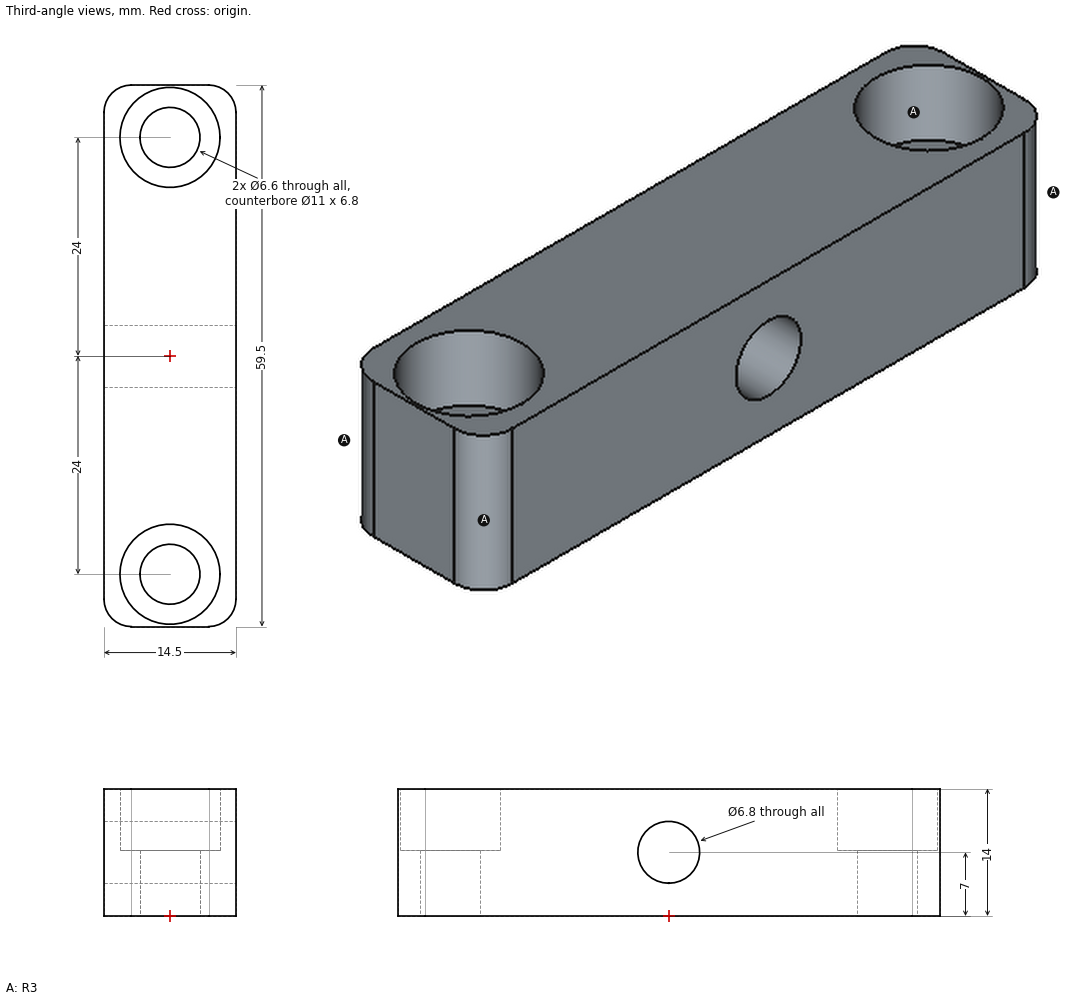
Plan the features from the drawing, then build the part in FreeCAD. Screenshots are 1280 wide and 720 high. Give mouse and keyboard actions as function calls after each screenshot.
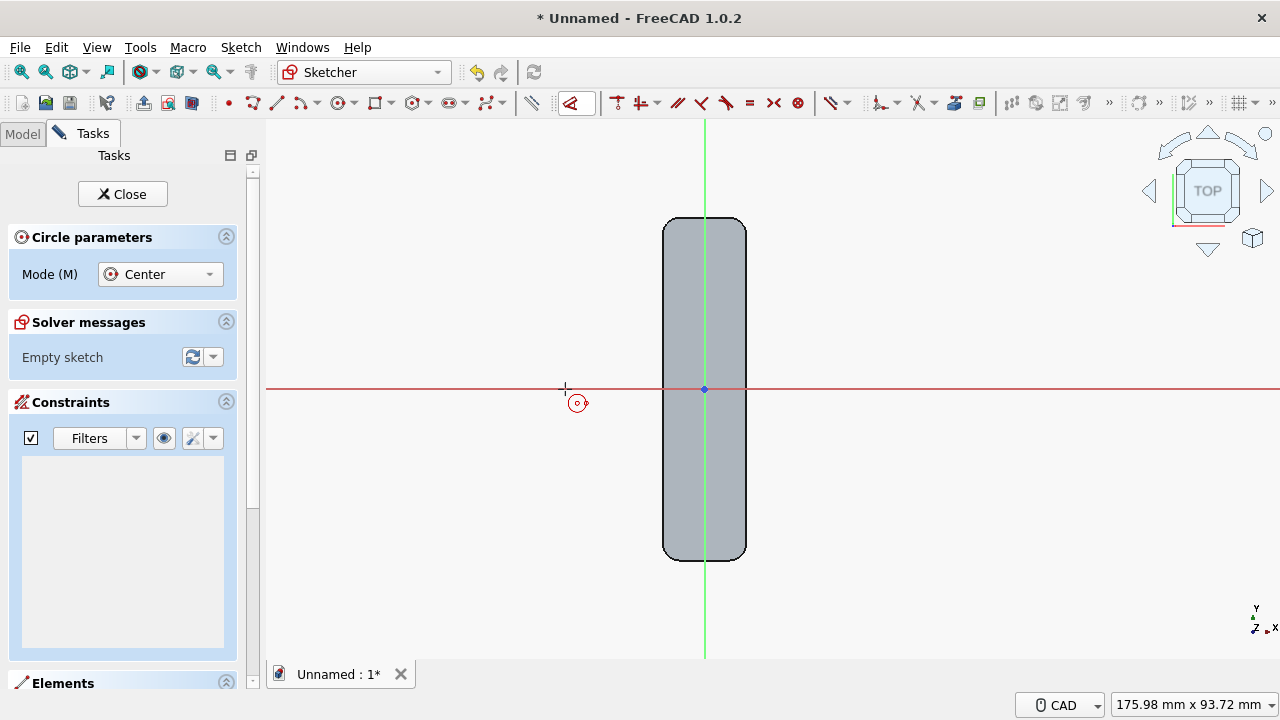
click(705, 251)
move(722, 244)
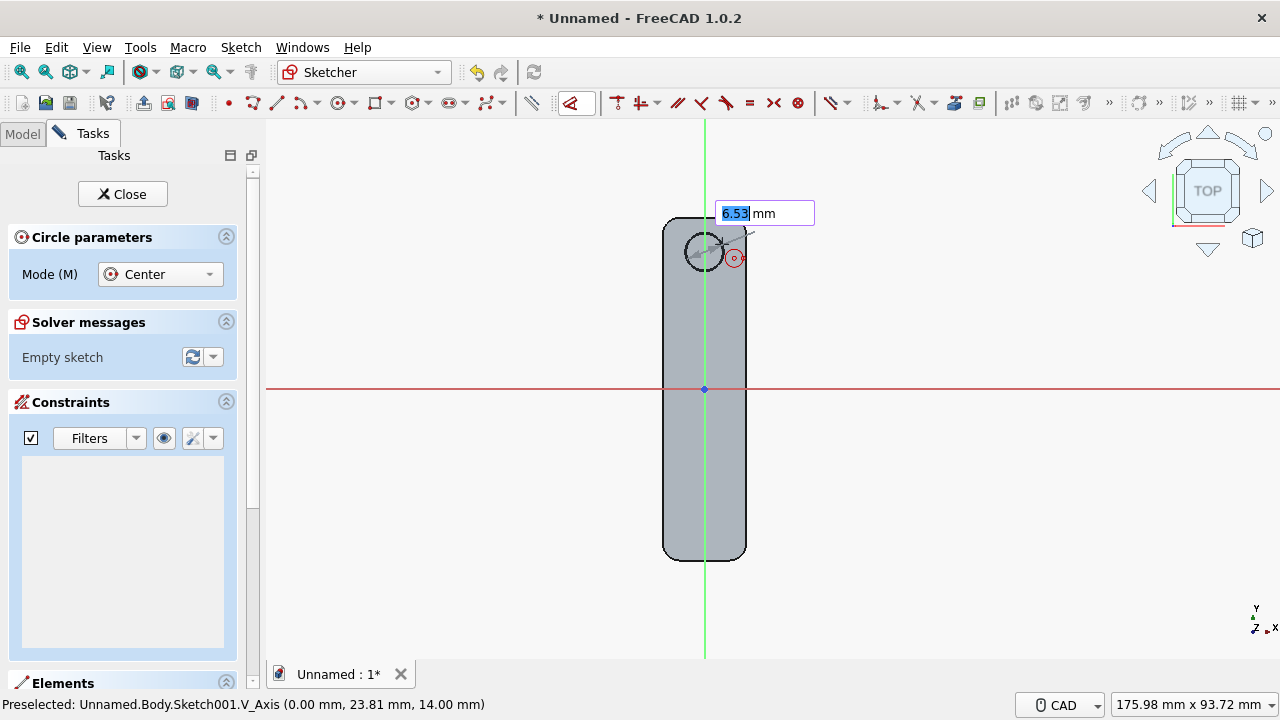
text(6.6)
key(Return)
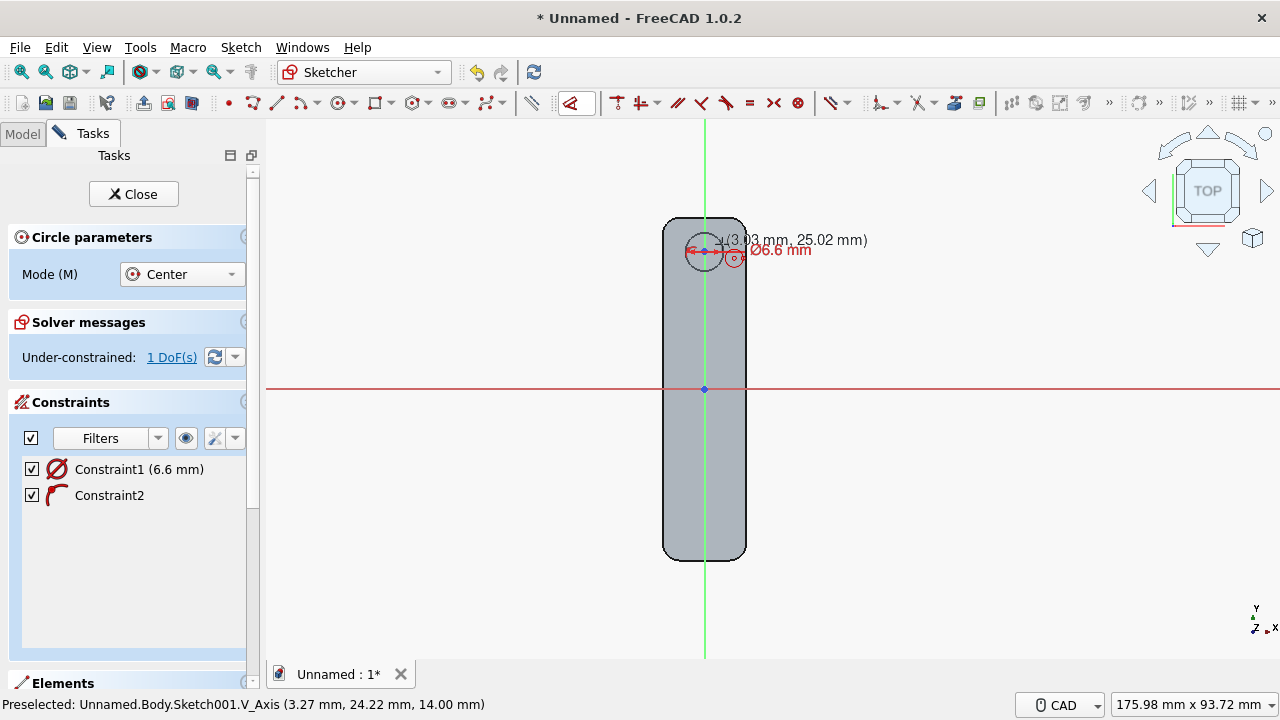
click(705, 527)
move(722, 521)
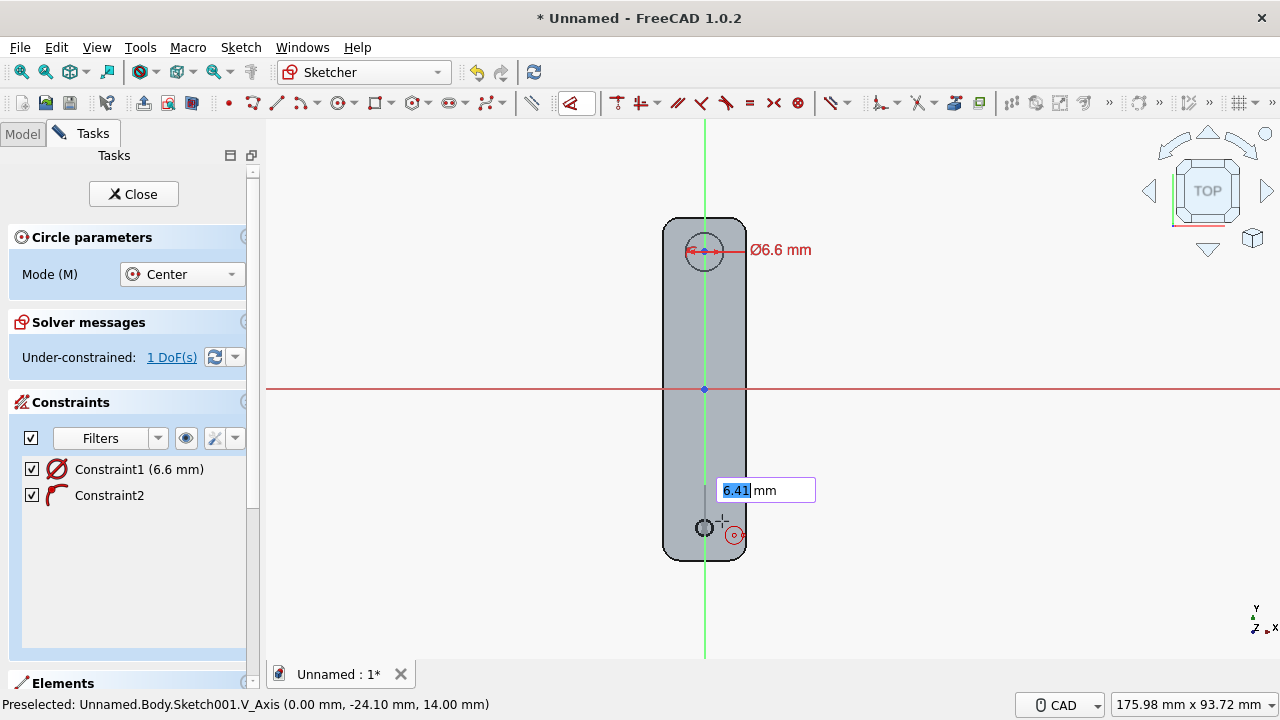
text(6.6)
key(Return)
key(Escape)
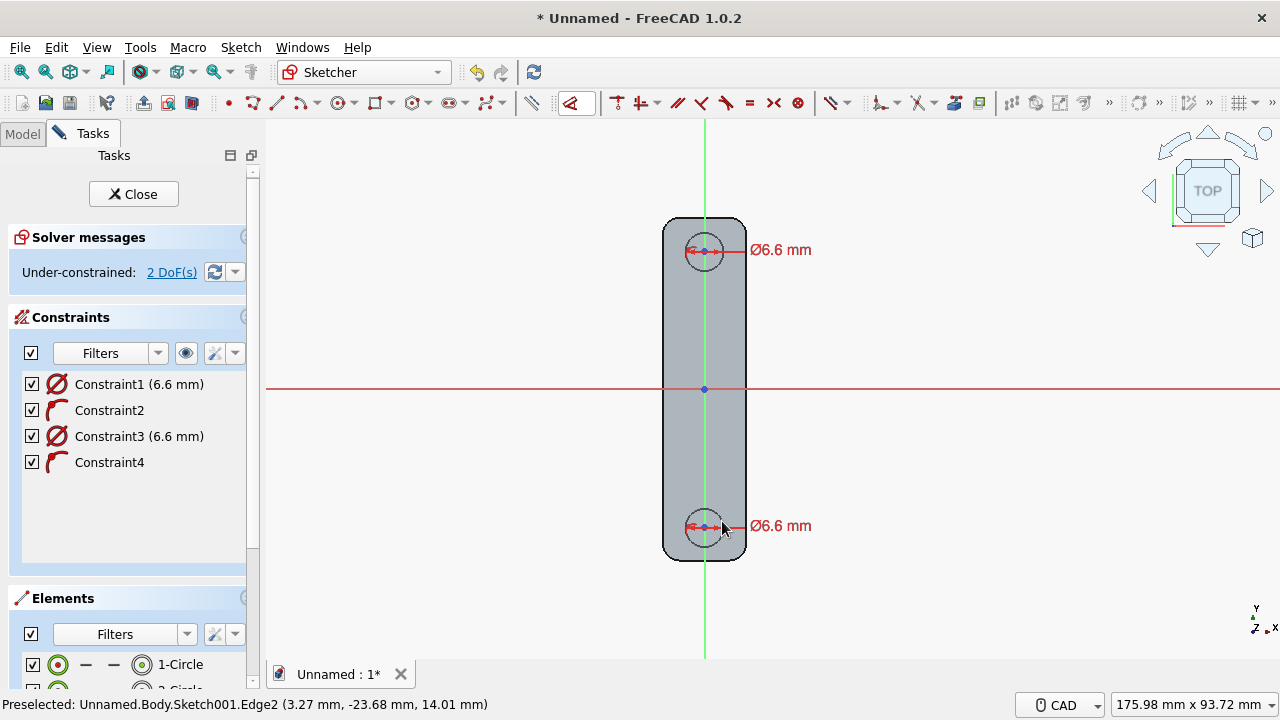
click(705, 252)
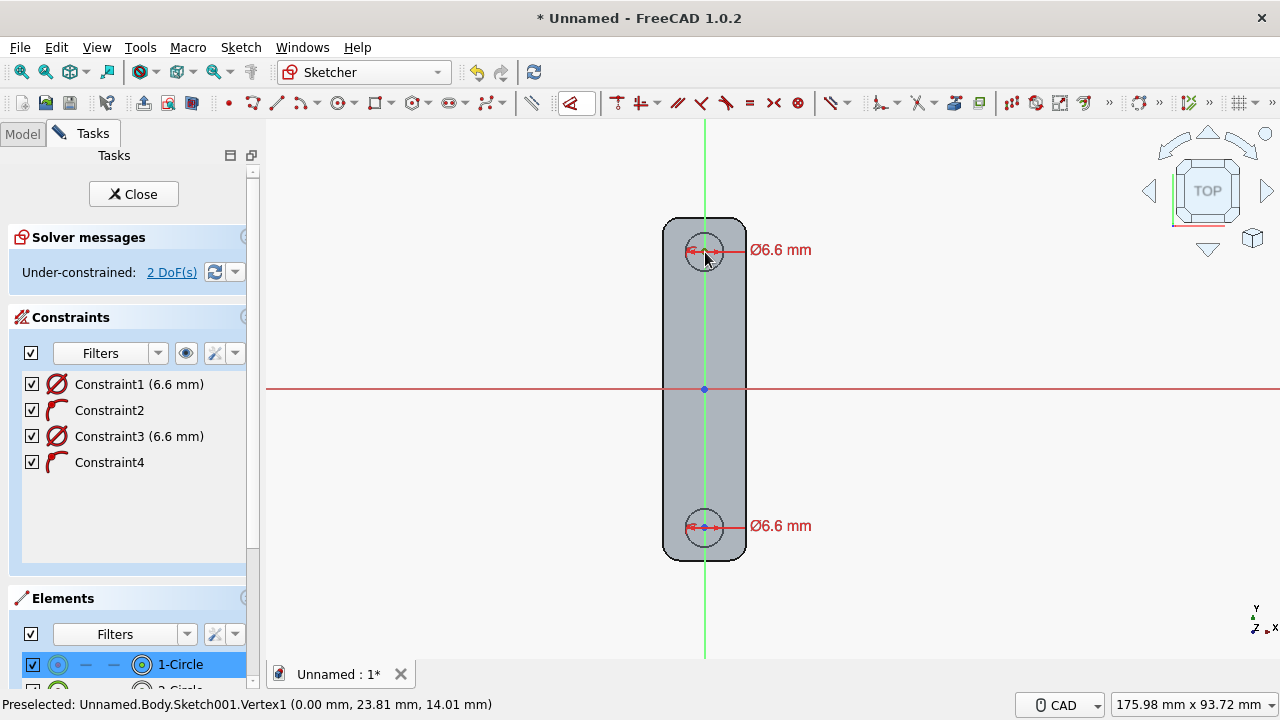
key(i)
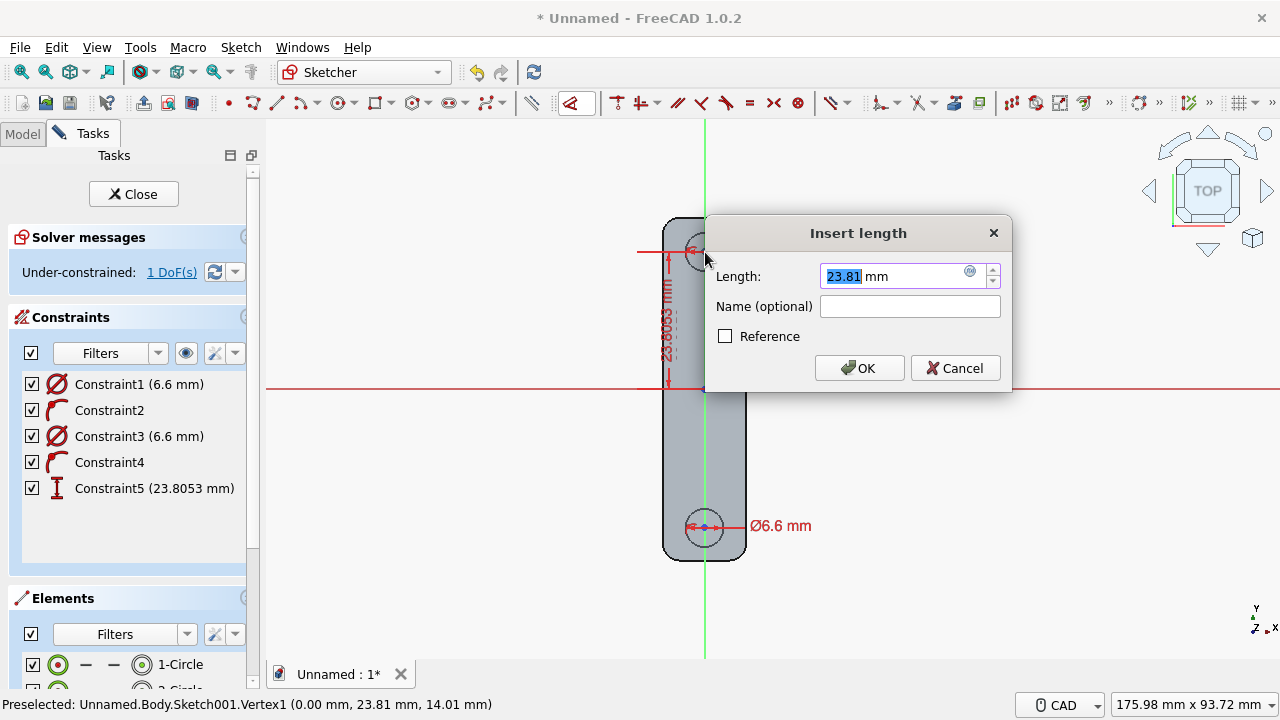
text(24)
key(Return)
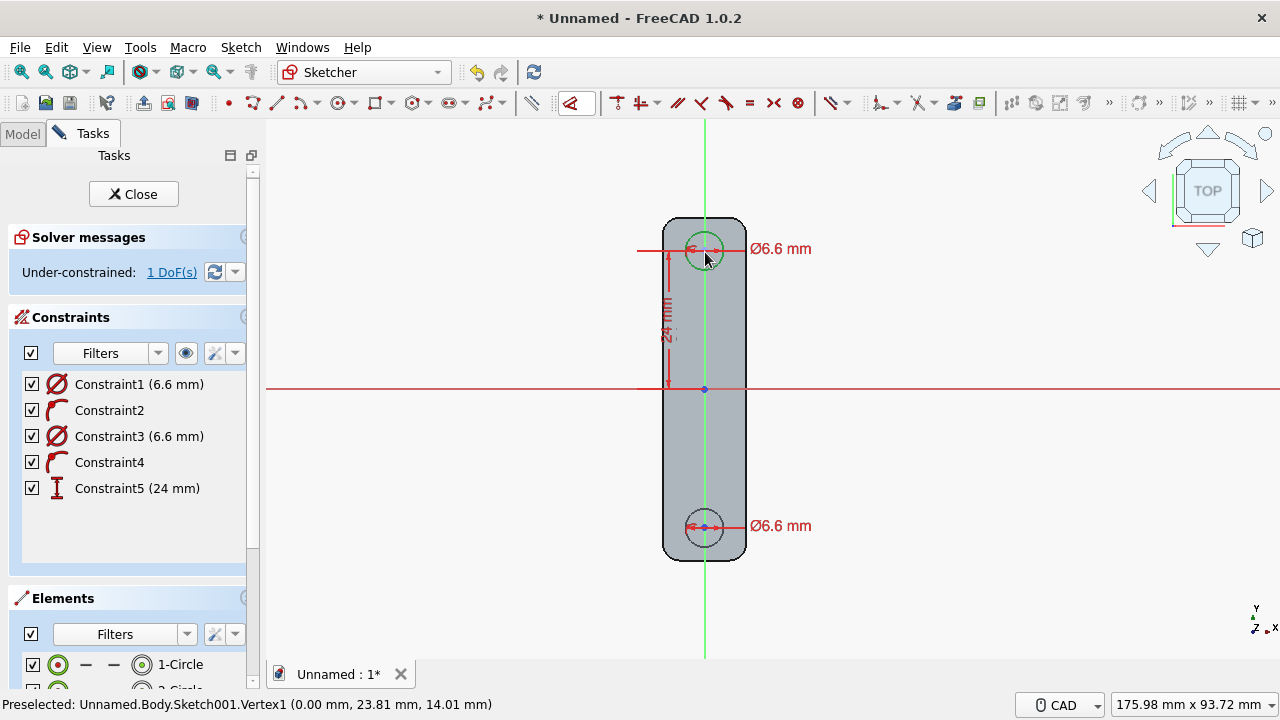
click(705, 528)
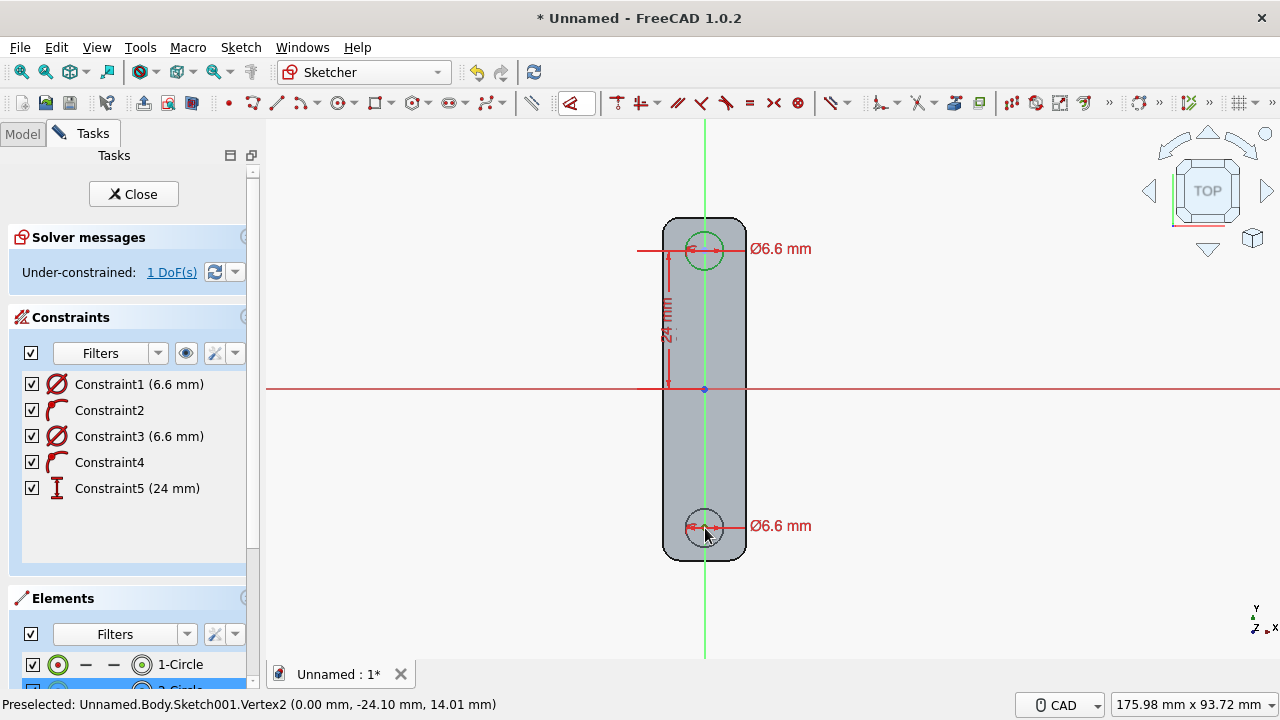
key(i)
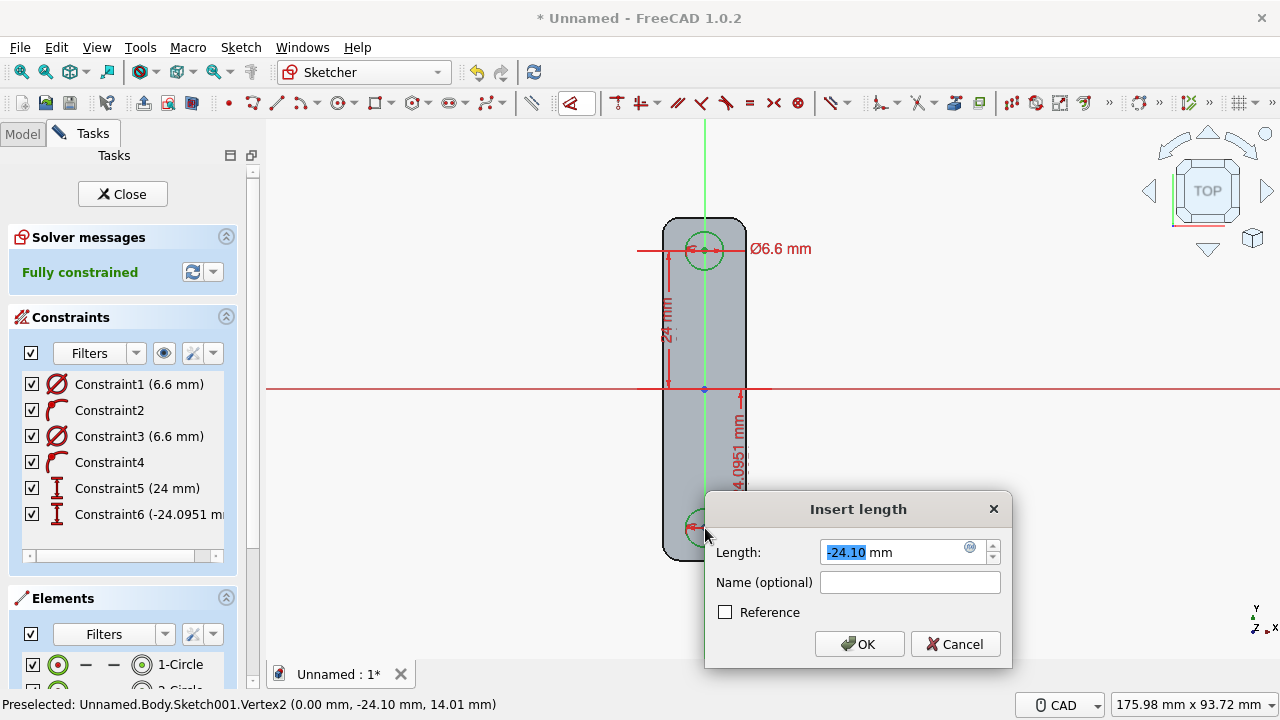
text(-24)
key(Return)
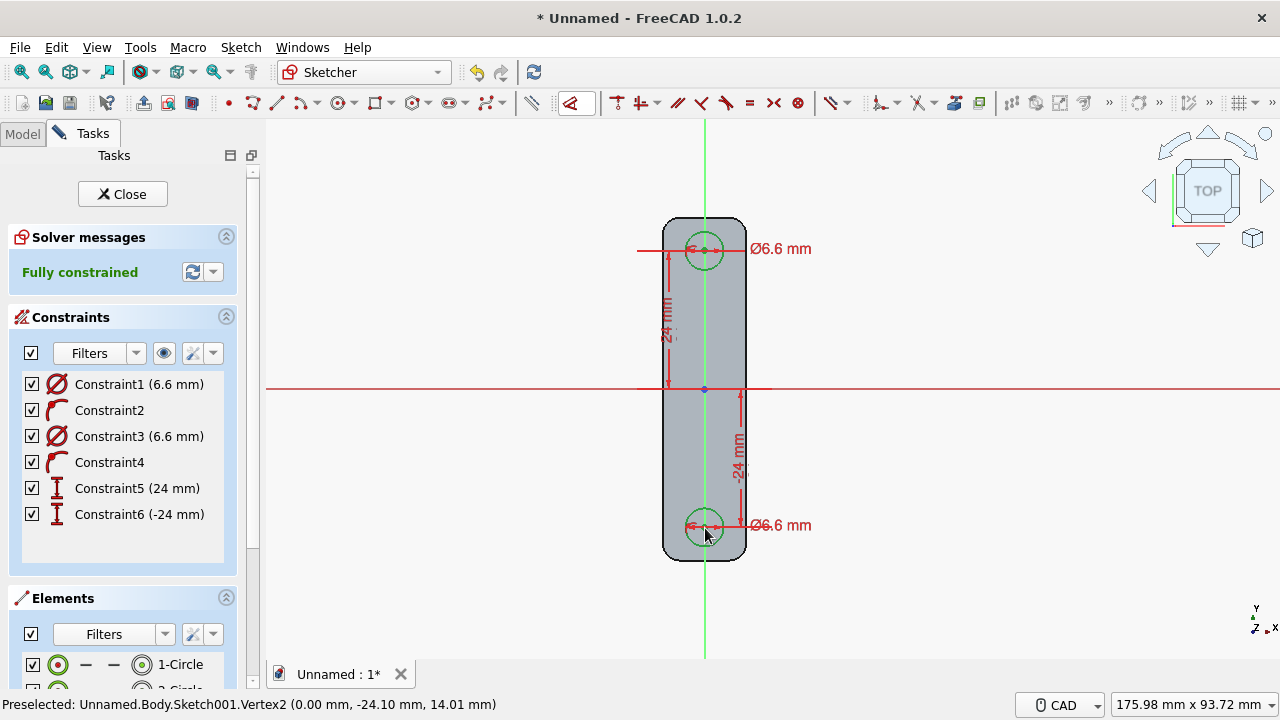
click(123, 194)